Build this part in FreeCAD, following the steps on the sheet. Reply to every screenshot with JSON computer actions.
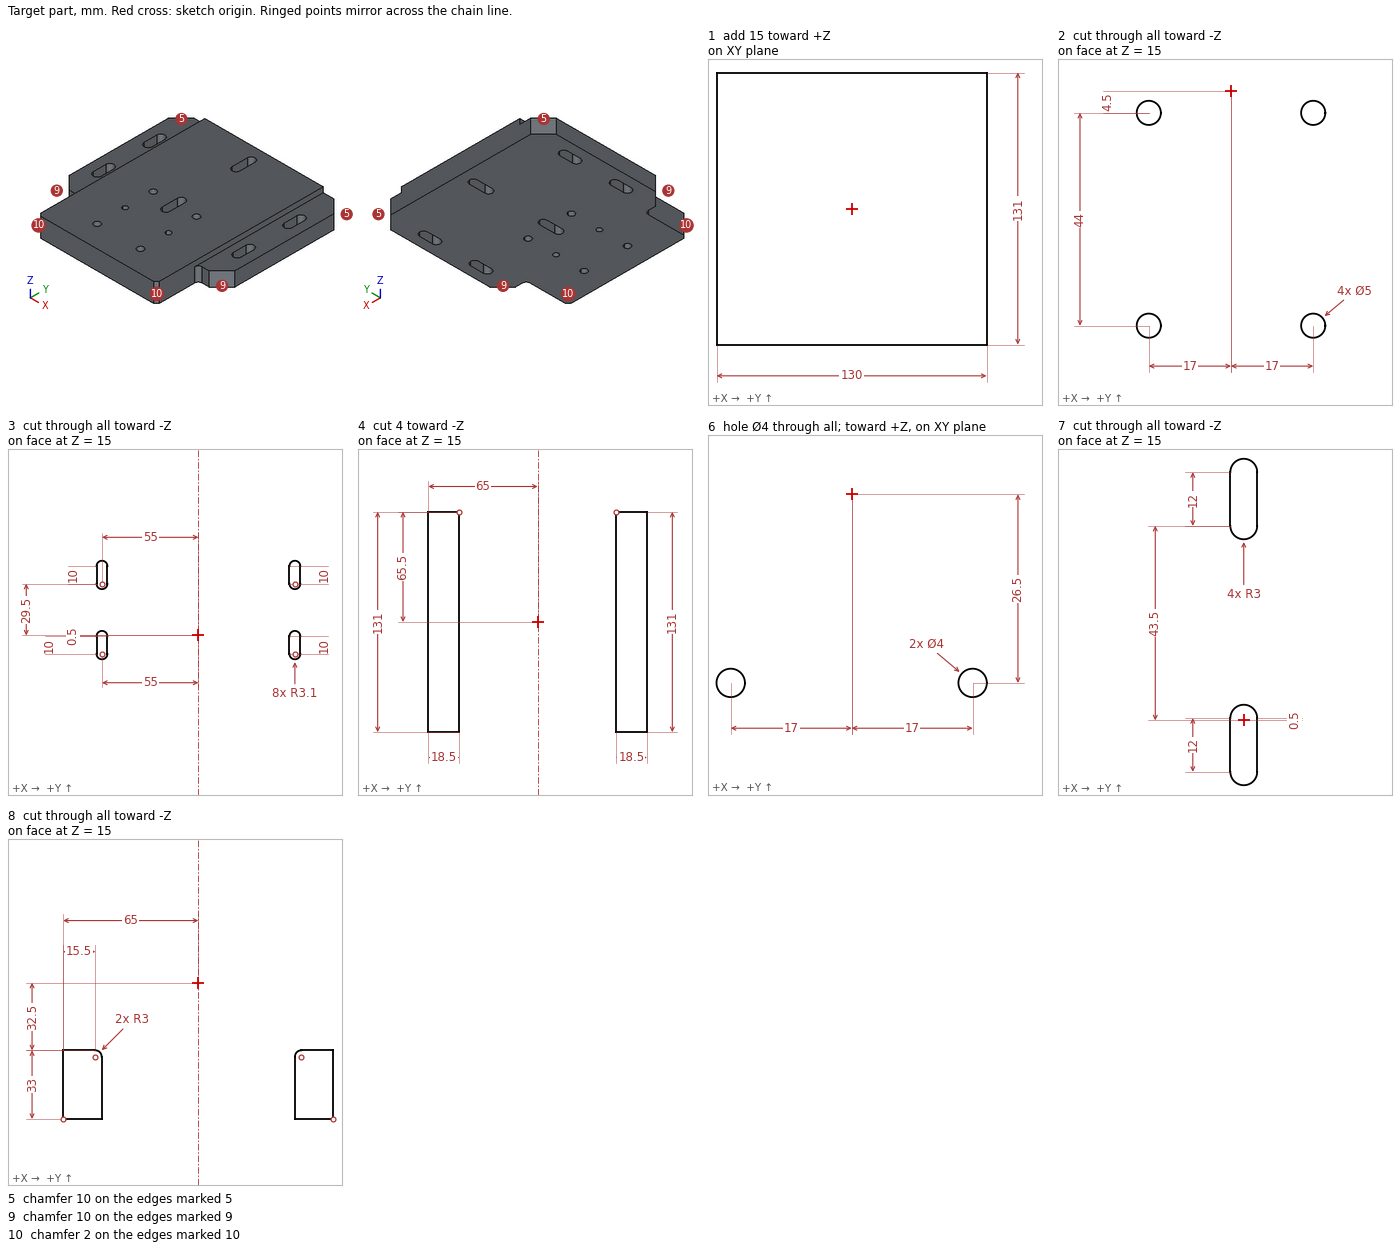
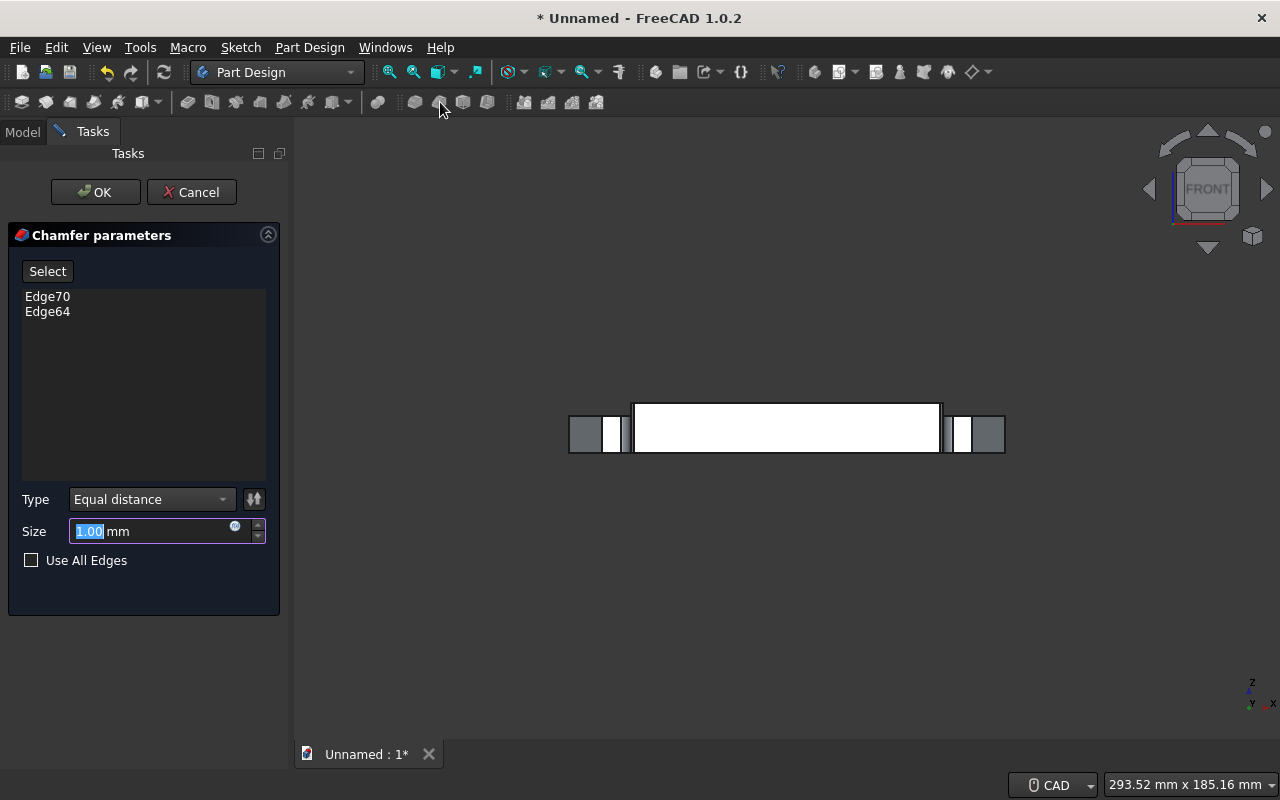
{"action": "type", "text": "2"}
{"action": "key", "text": "Tab"}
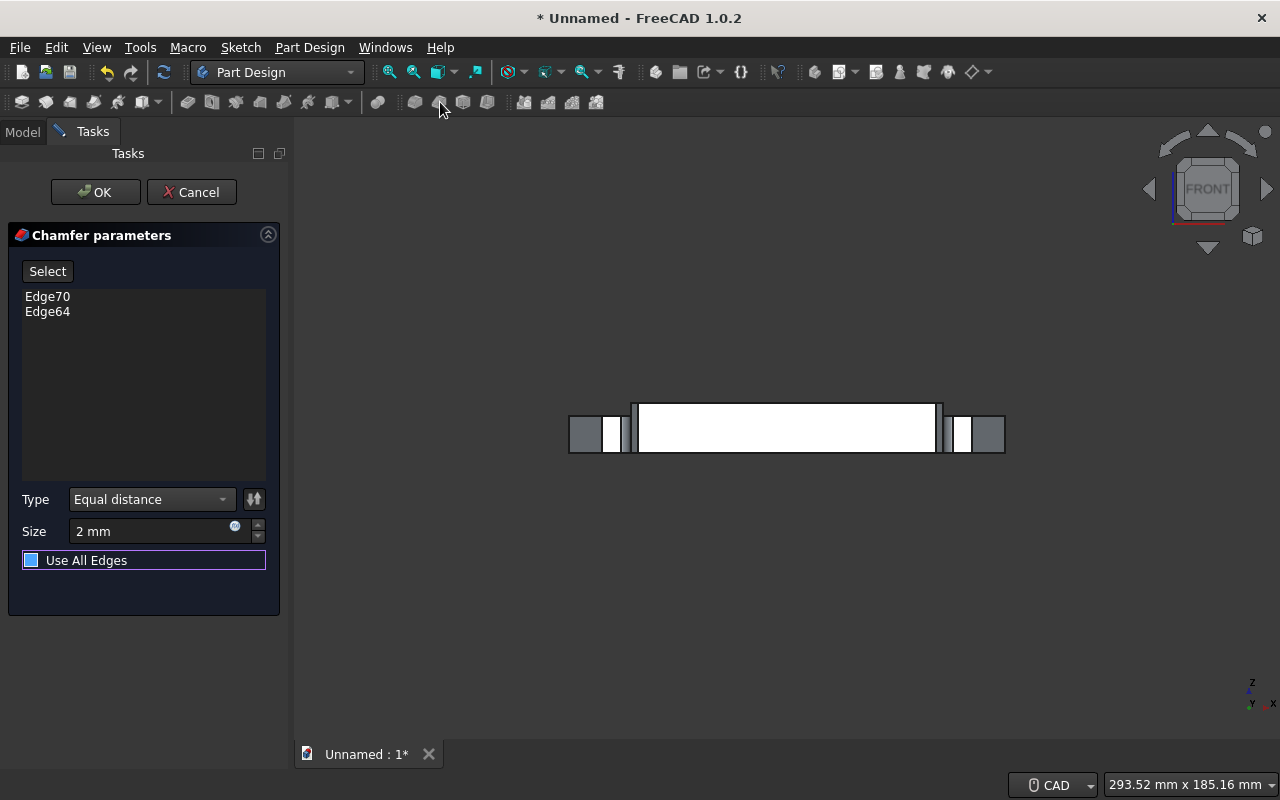
{"action": "left_click", "coordinate": [96, 192]}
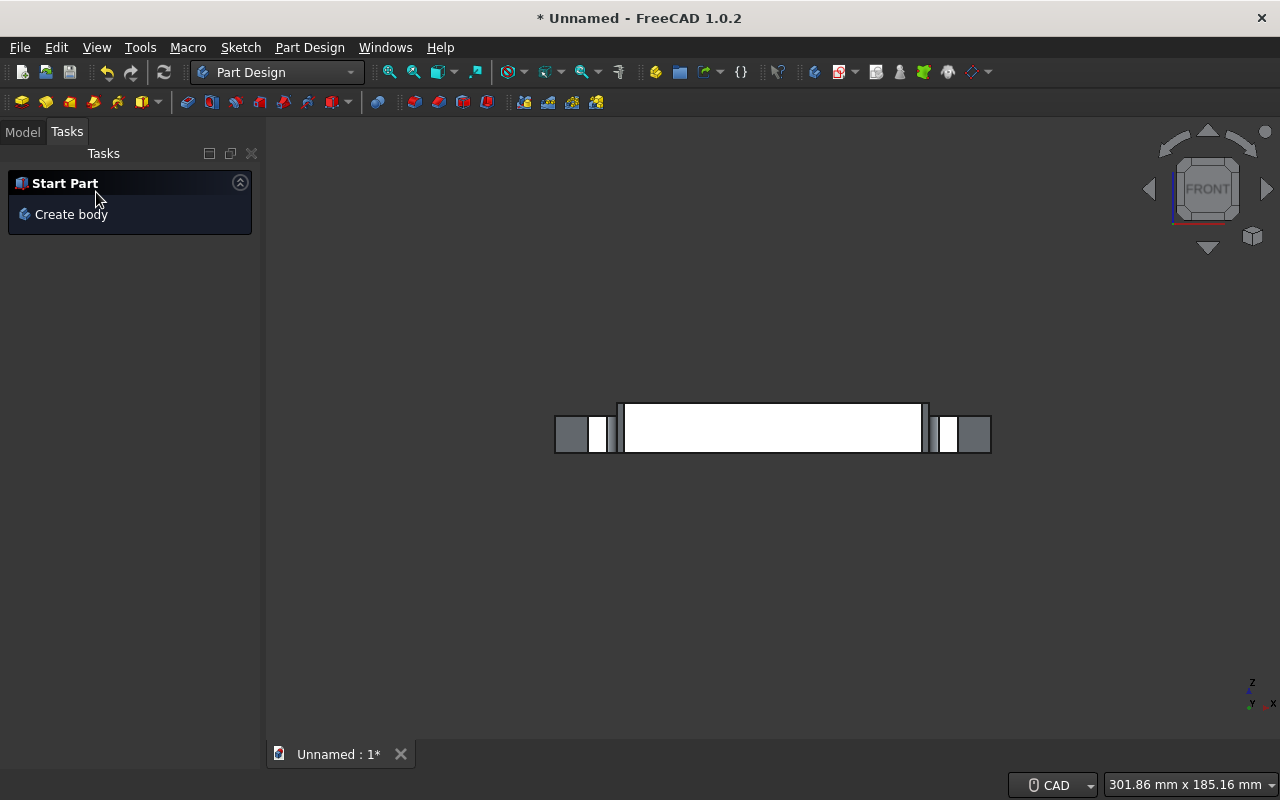
{"action": "key", "text": "0"}